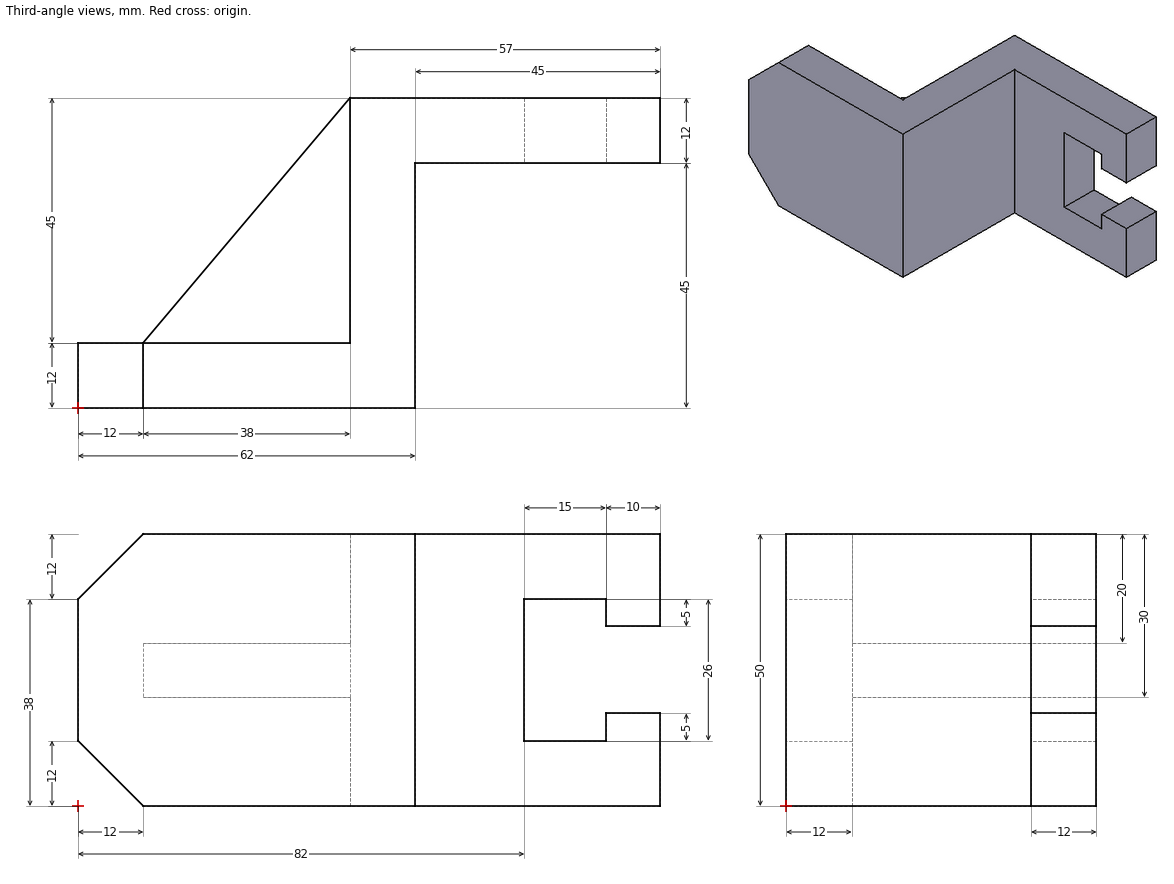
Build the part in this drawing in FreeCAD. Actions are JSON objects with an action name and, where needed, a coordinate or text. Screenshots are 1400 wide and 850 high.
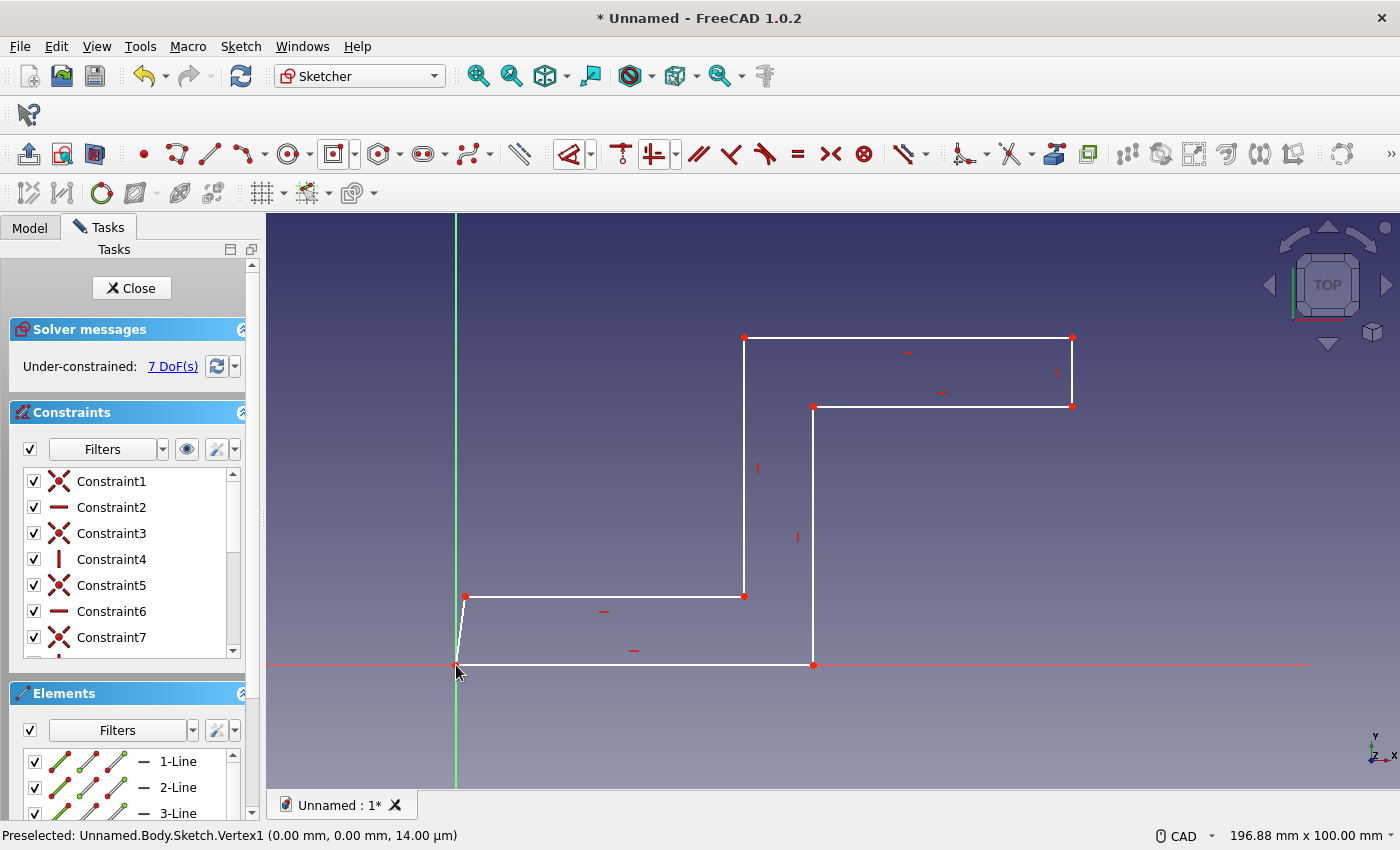
{"action": "left_click", "coordinate": [459, 645]}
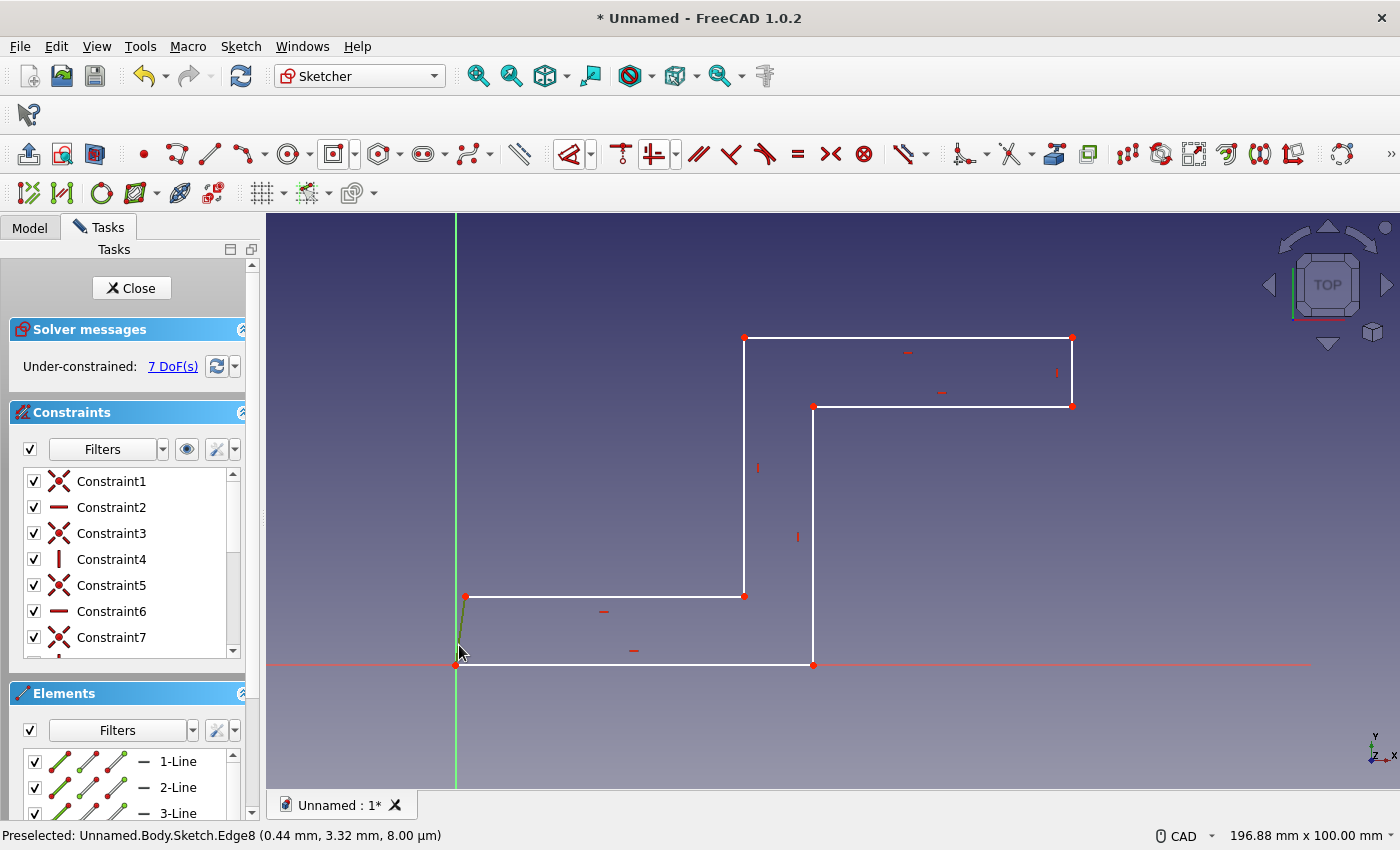
{"action": "left_click", "coordinate": [676, 154]}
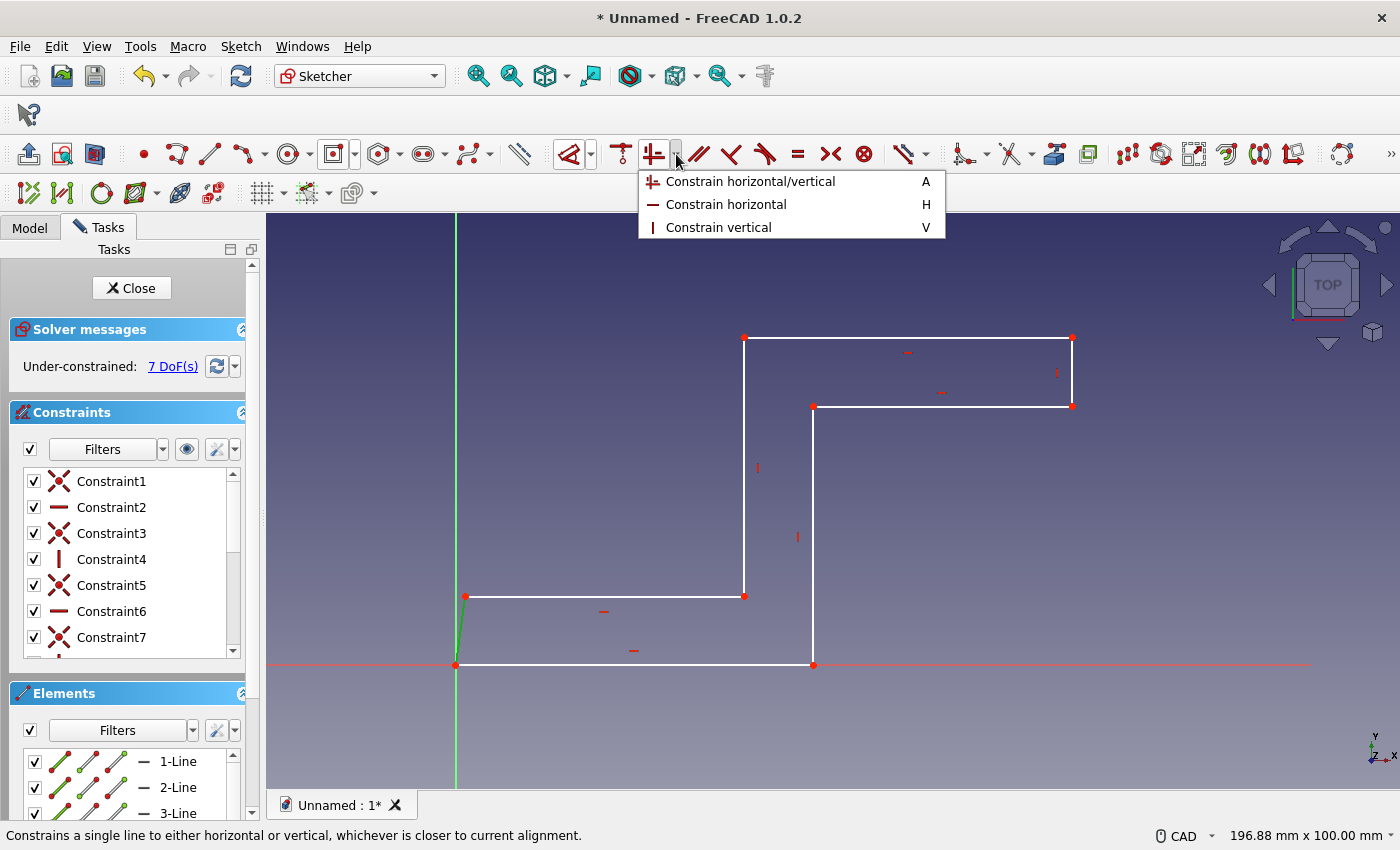
{"action": "left_click", "coordinate": [792, 228]}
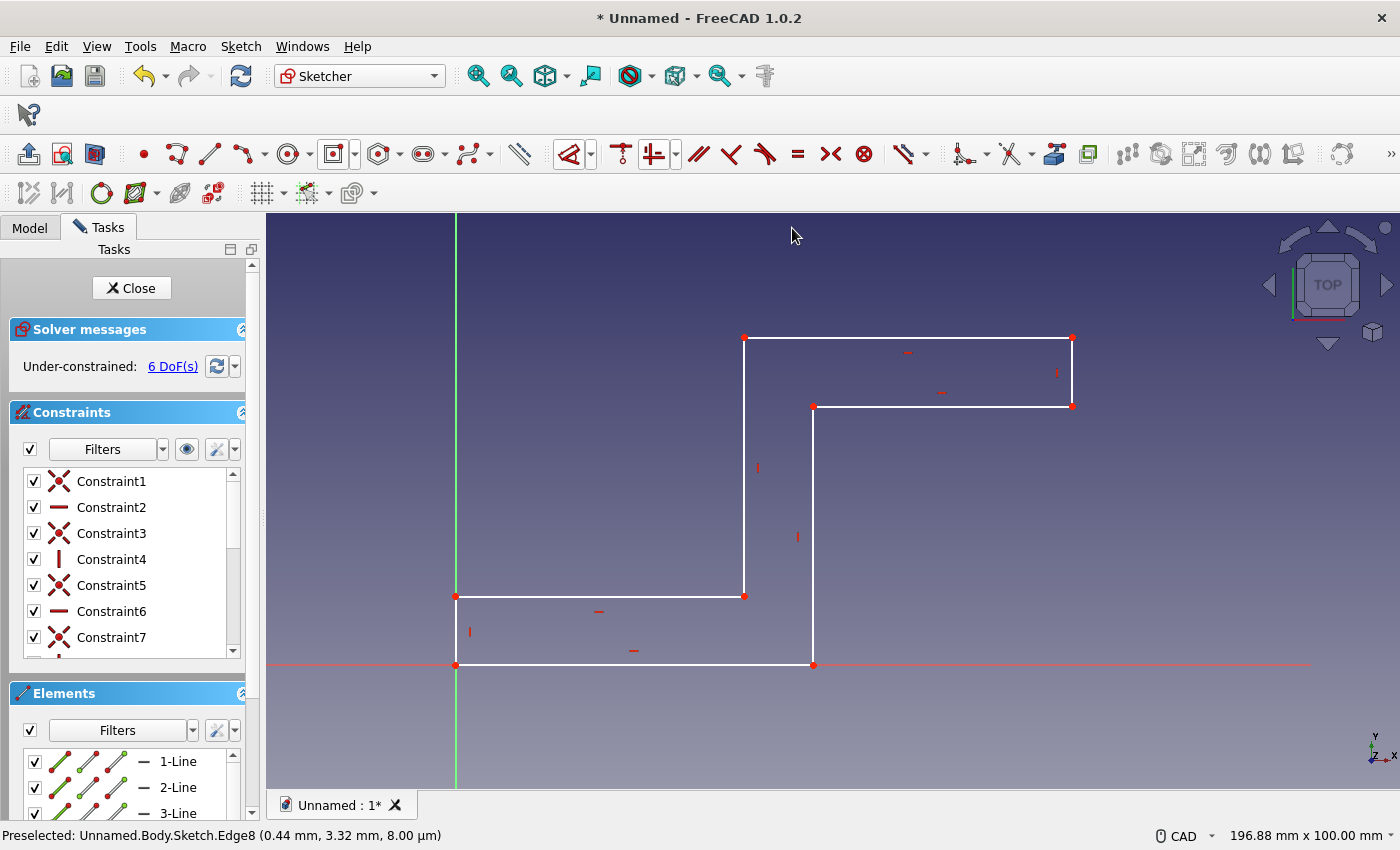
{"action": "left_click", "coordinate": [568, 154]}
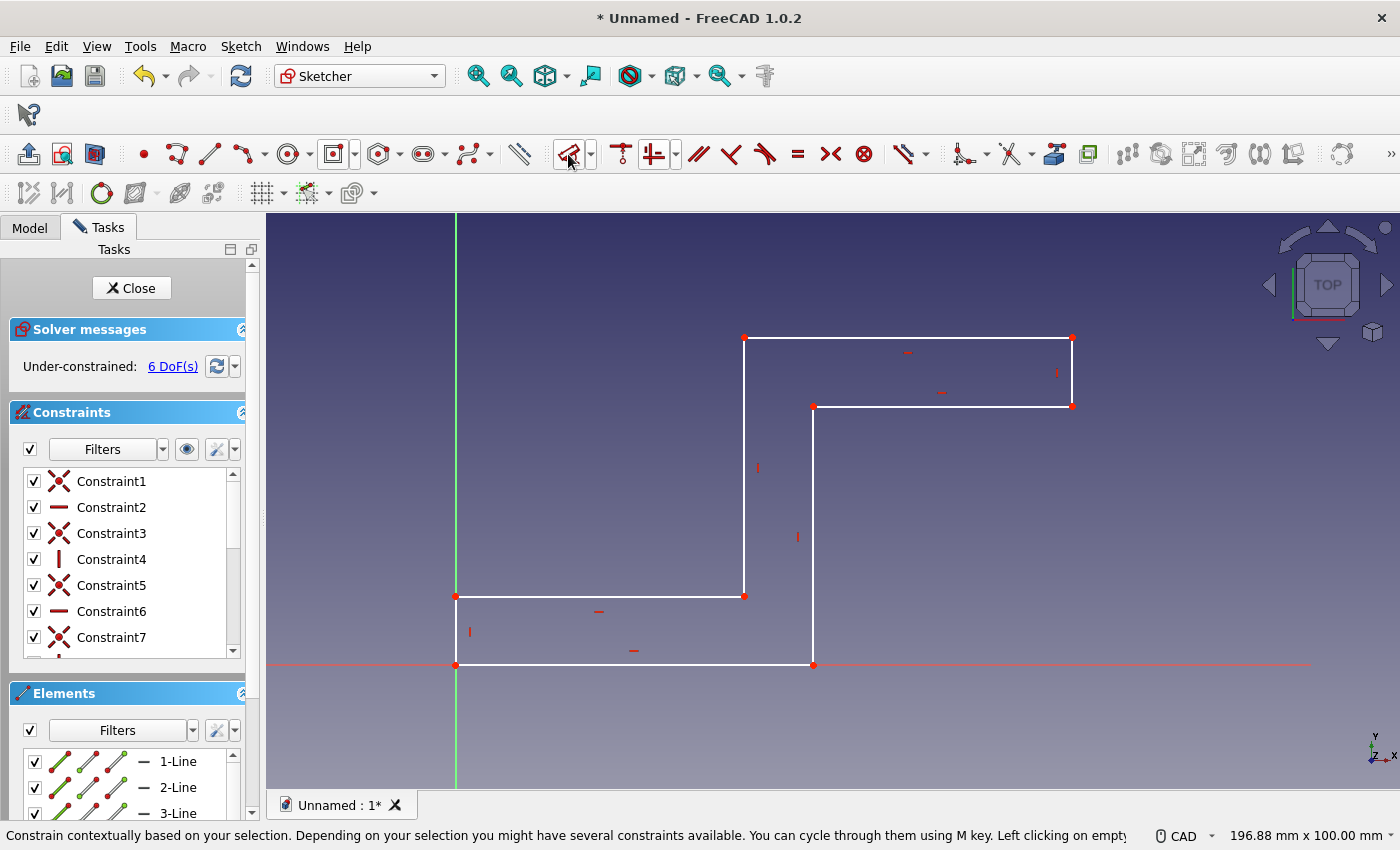
{"action": "left_click", "coordinate": [563, 665]}
{"action": "left_click", "coordinate": [634, 699]}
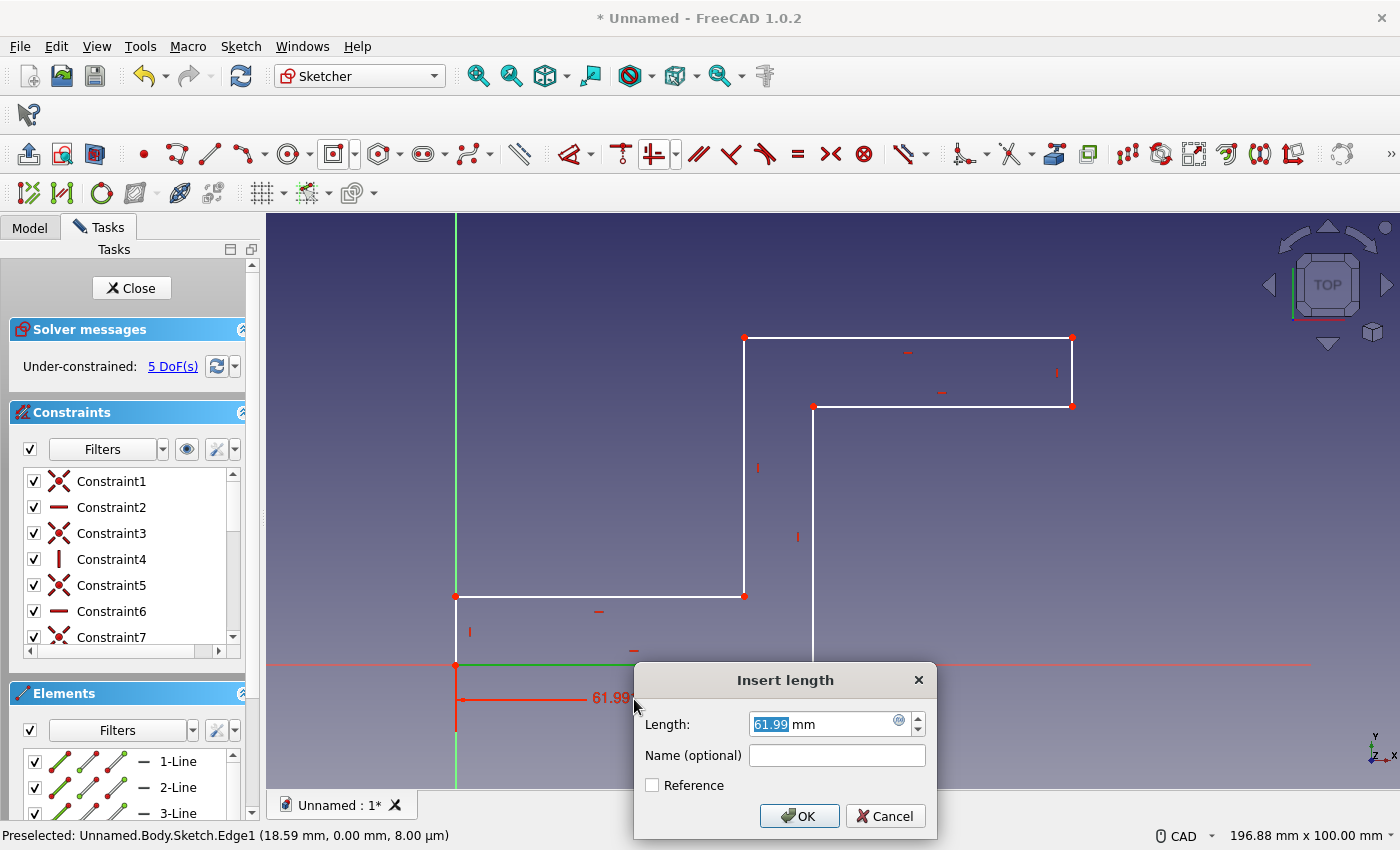
{"action": "type", "text": "62"}
{"action": "key", "text": "Return"}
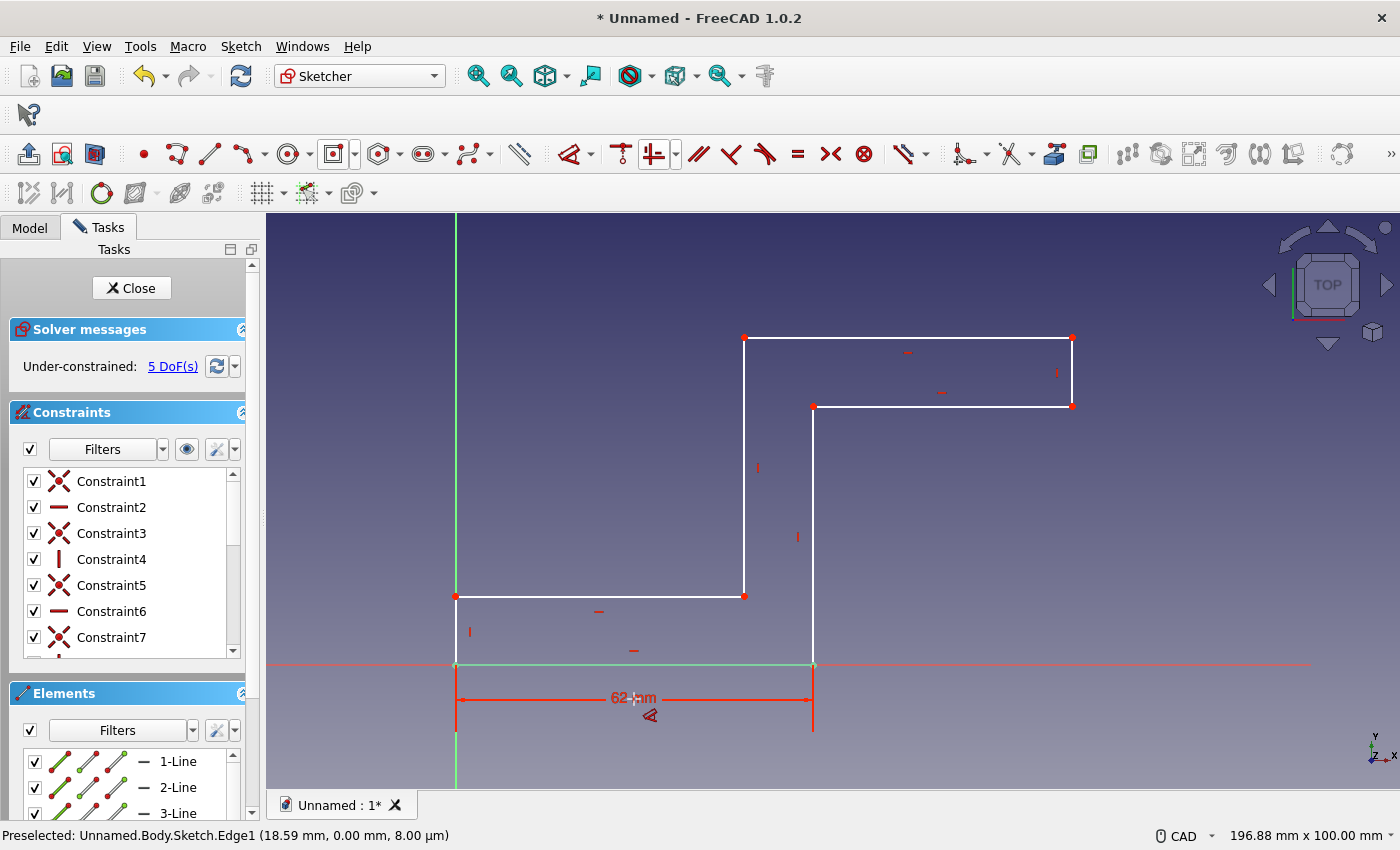
{"action": "left_click", "coordinate": [813, 588]}
{"action": "left_click", "coordinate": [847, 536]}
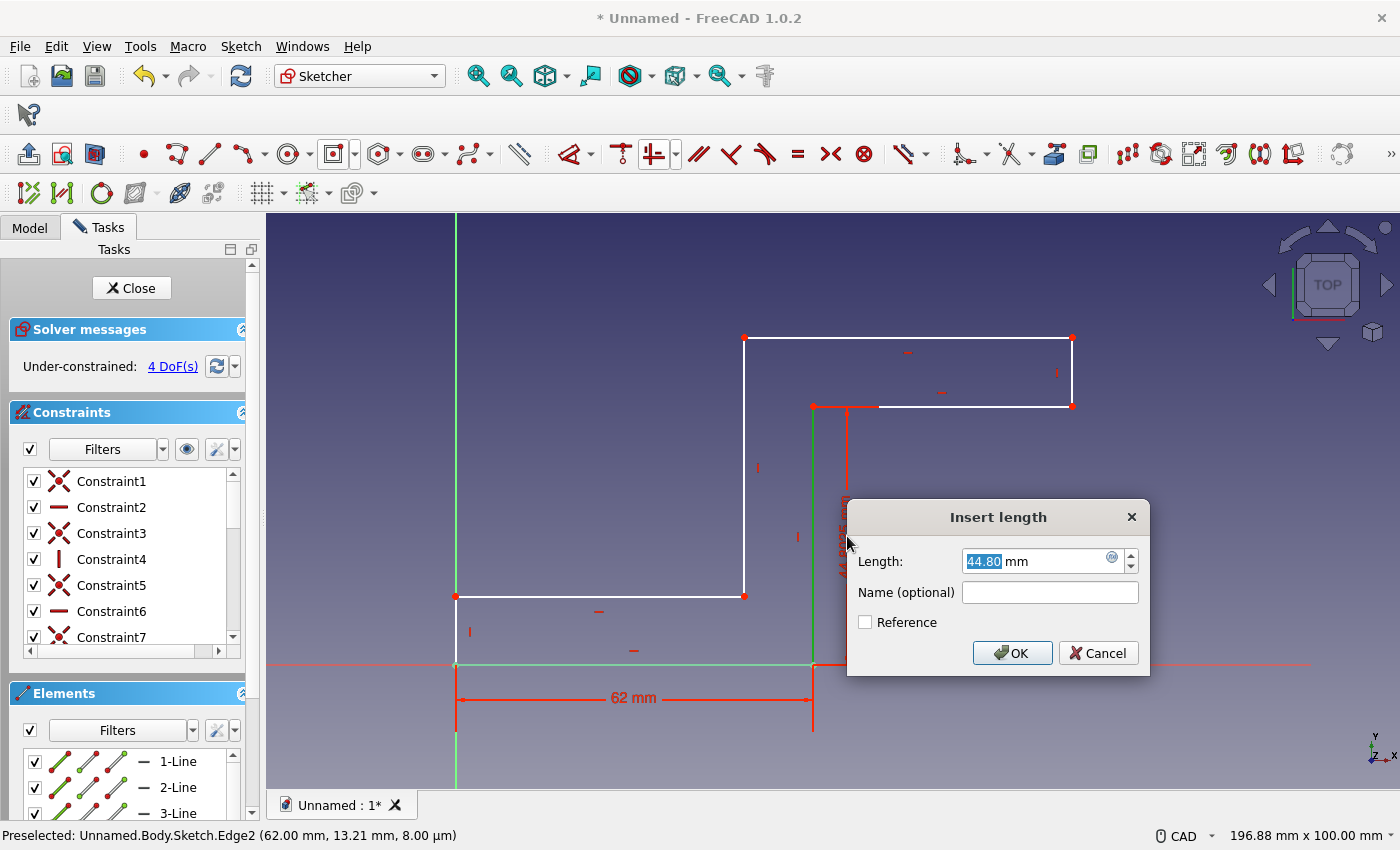
{"action": "type", "text": "45"}
{"action": "key", "text": "Return"}